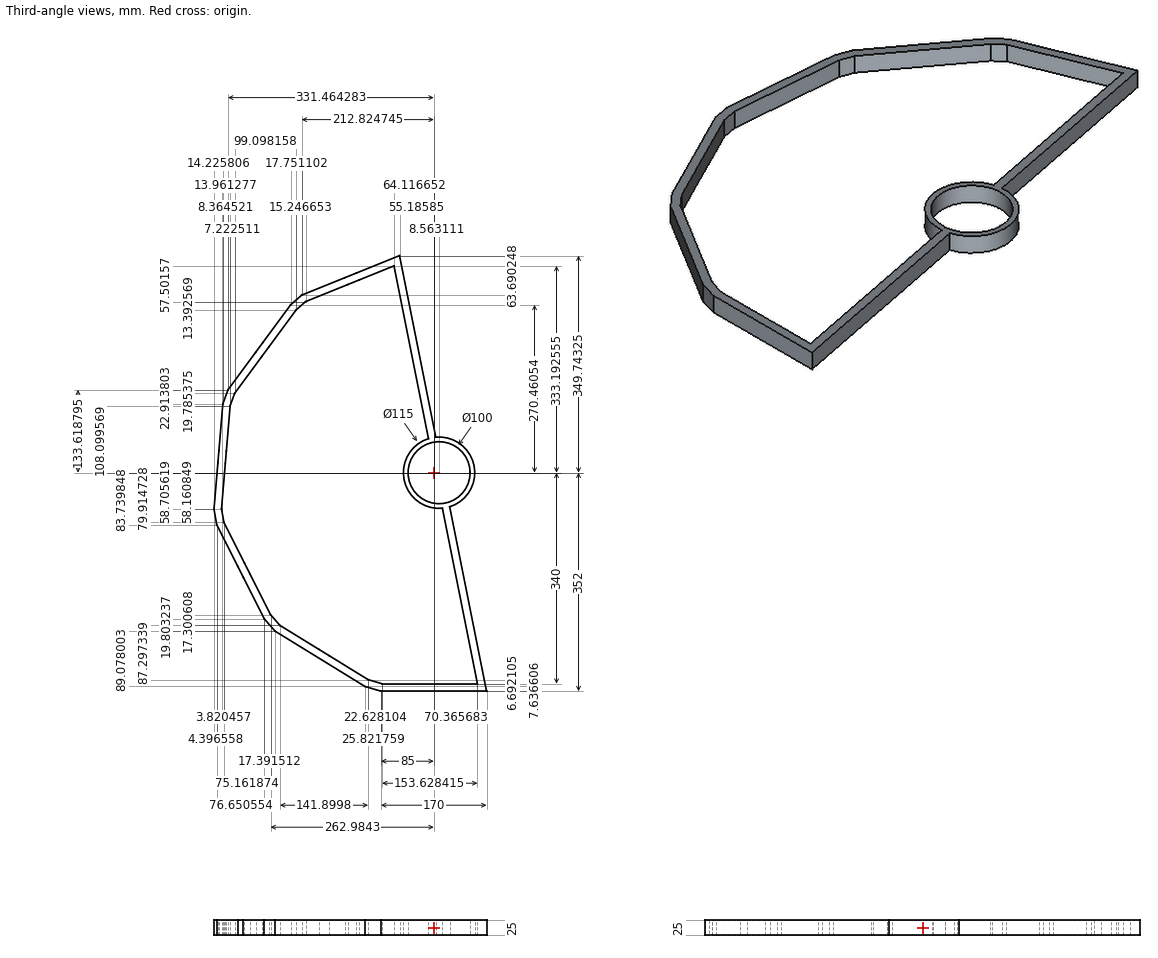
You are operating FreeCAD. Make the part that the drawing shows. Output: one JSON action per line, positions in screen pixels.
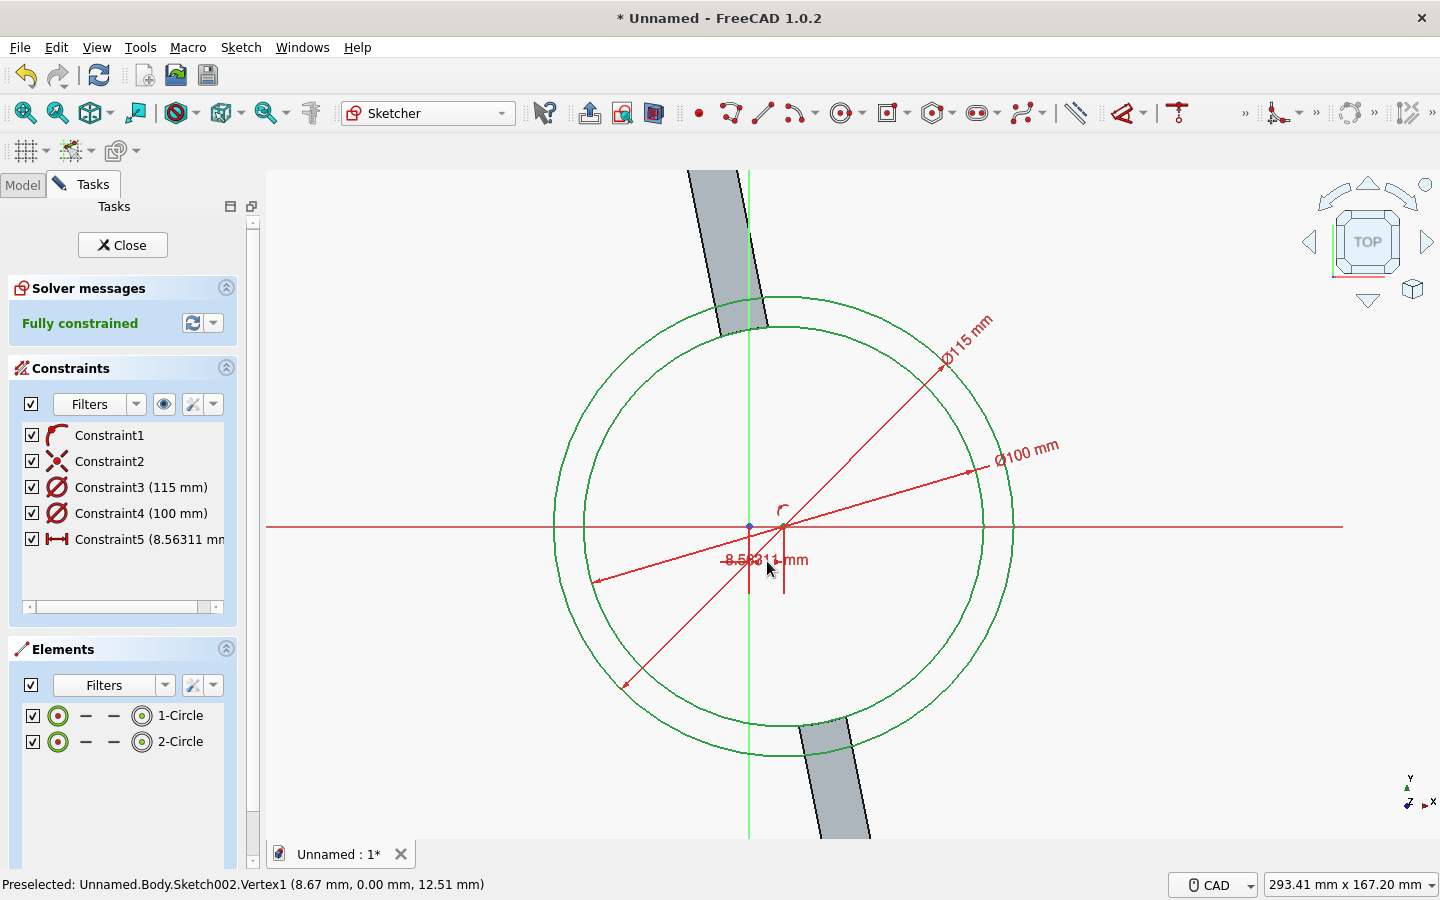
{"action": "left_click", "coordinate": [123, 245]}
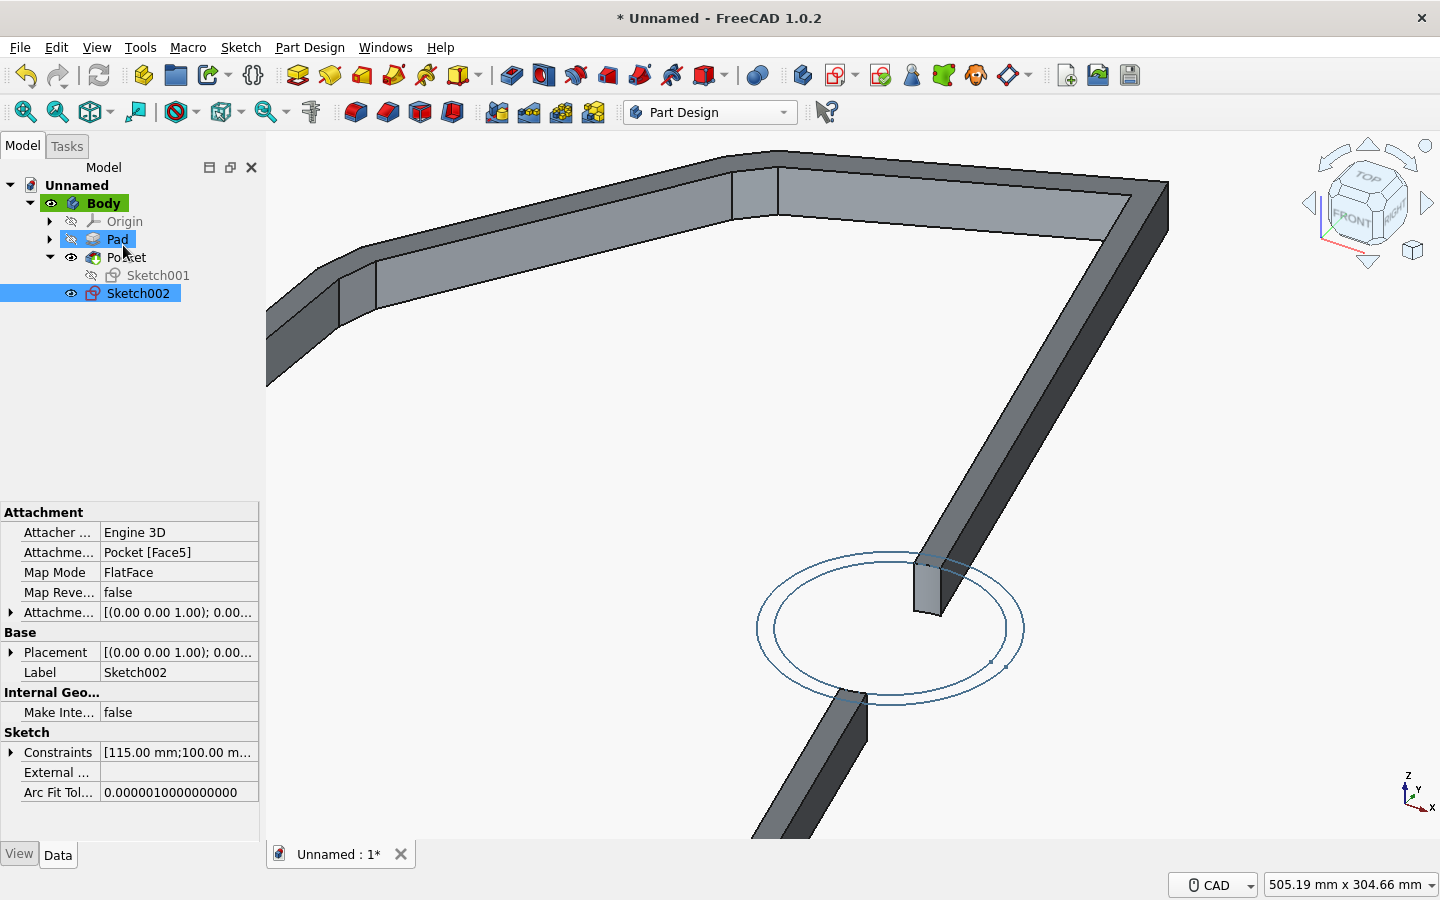
{"action": "left_click", "coordinate": [298, 76]}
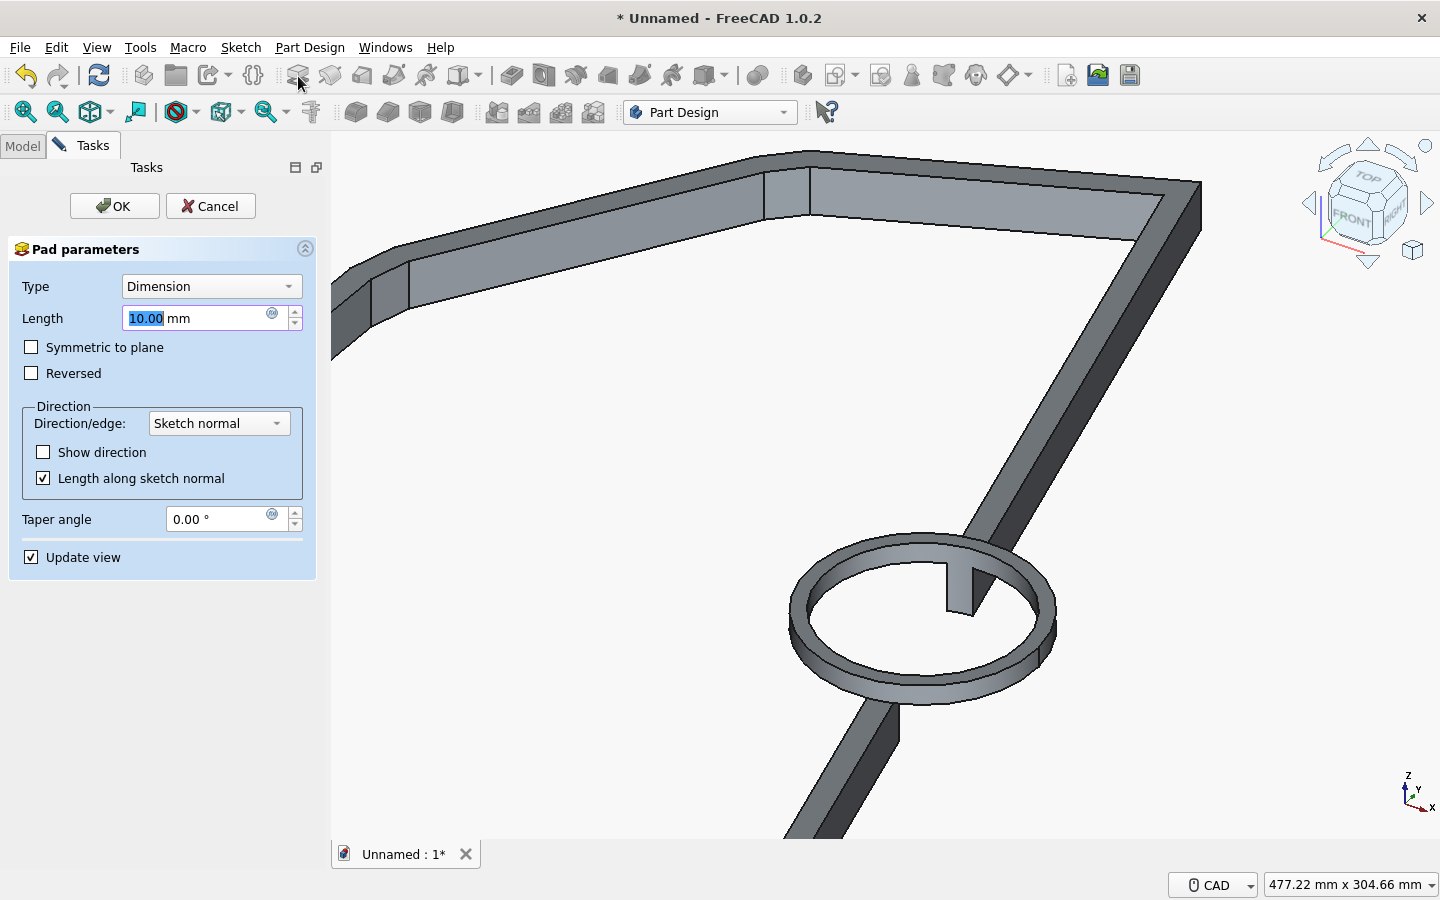
{"action": "type", "text": "25"}
{"action": "key", "text": "Tab"}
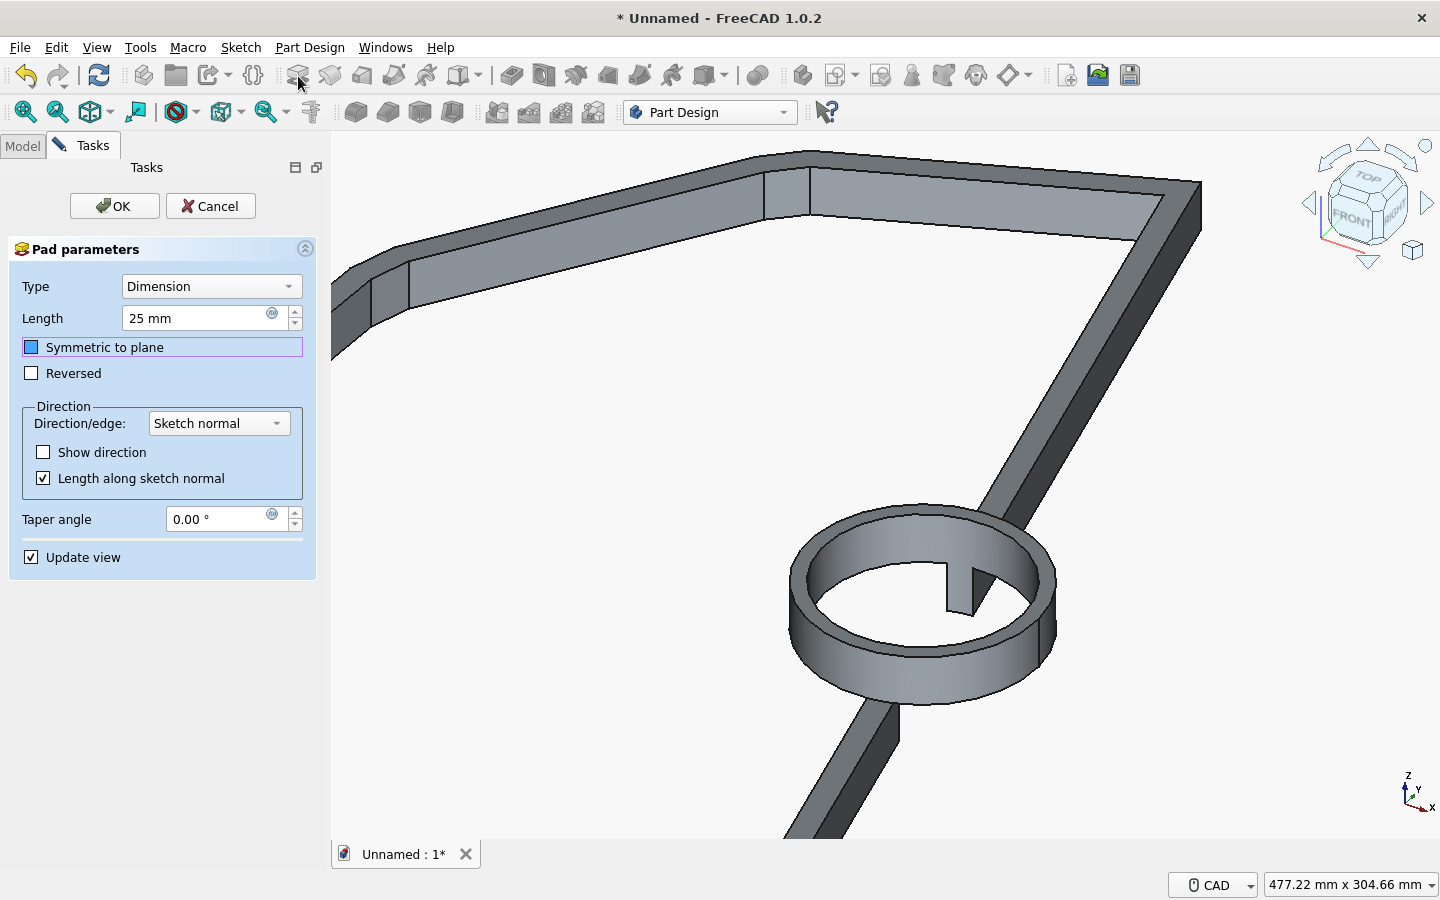
{"action": "left_click", "coordinate": [30, 373]}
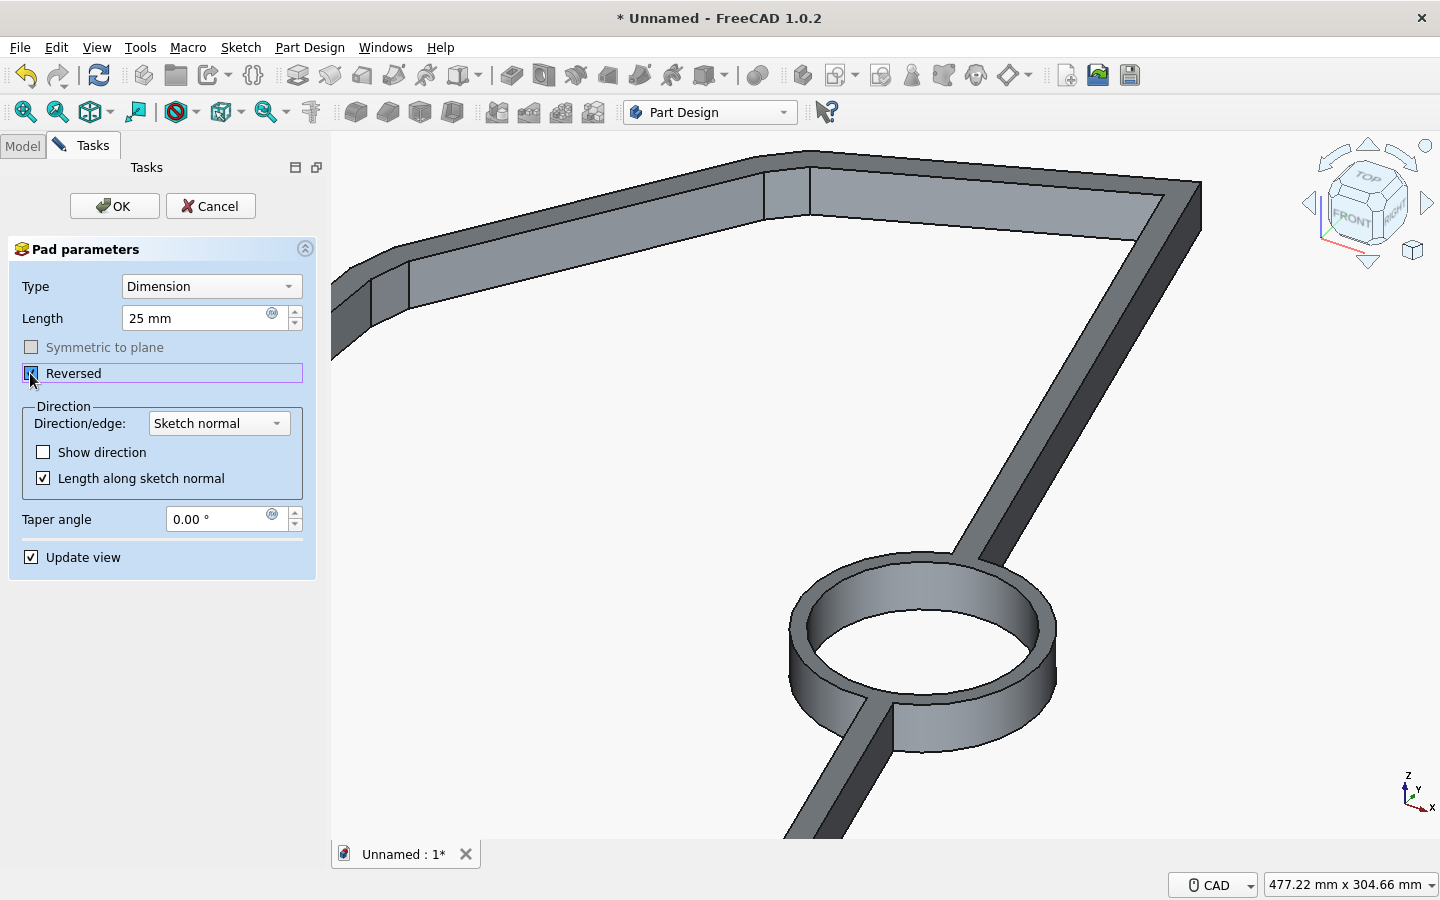
{"action": "left_click", "coordinate": [115, 206]}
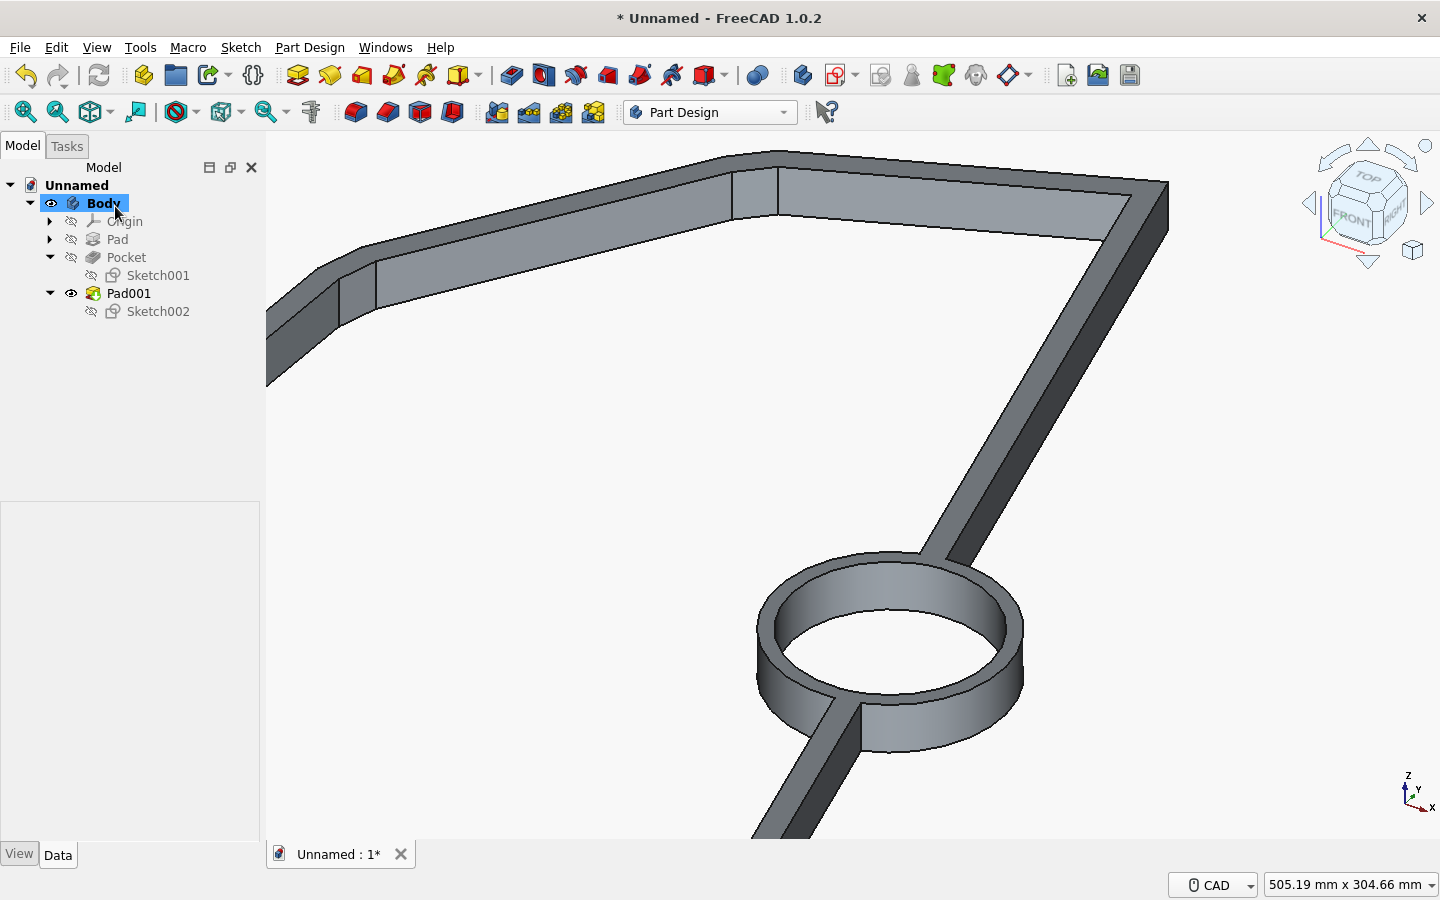
{"action": "key", "text": "0"}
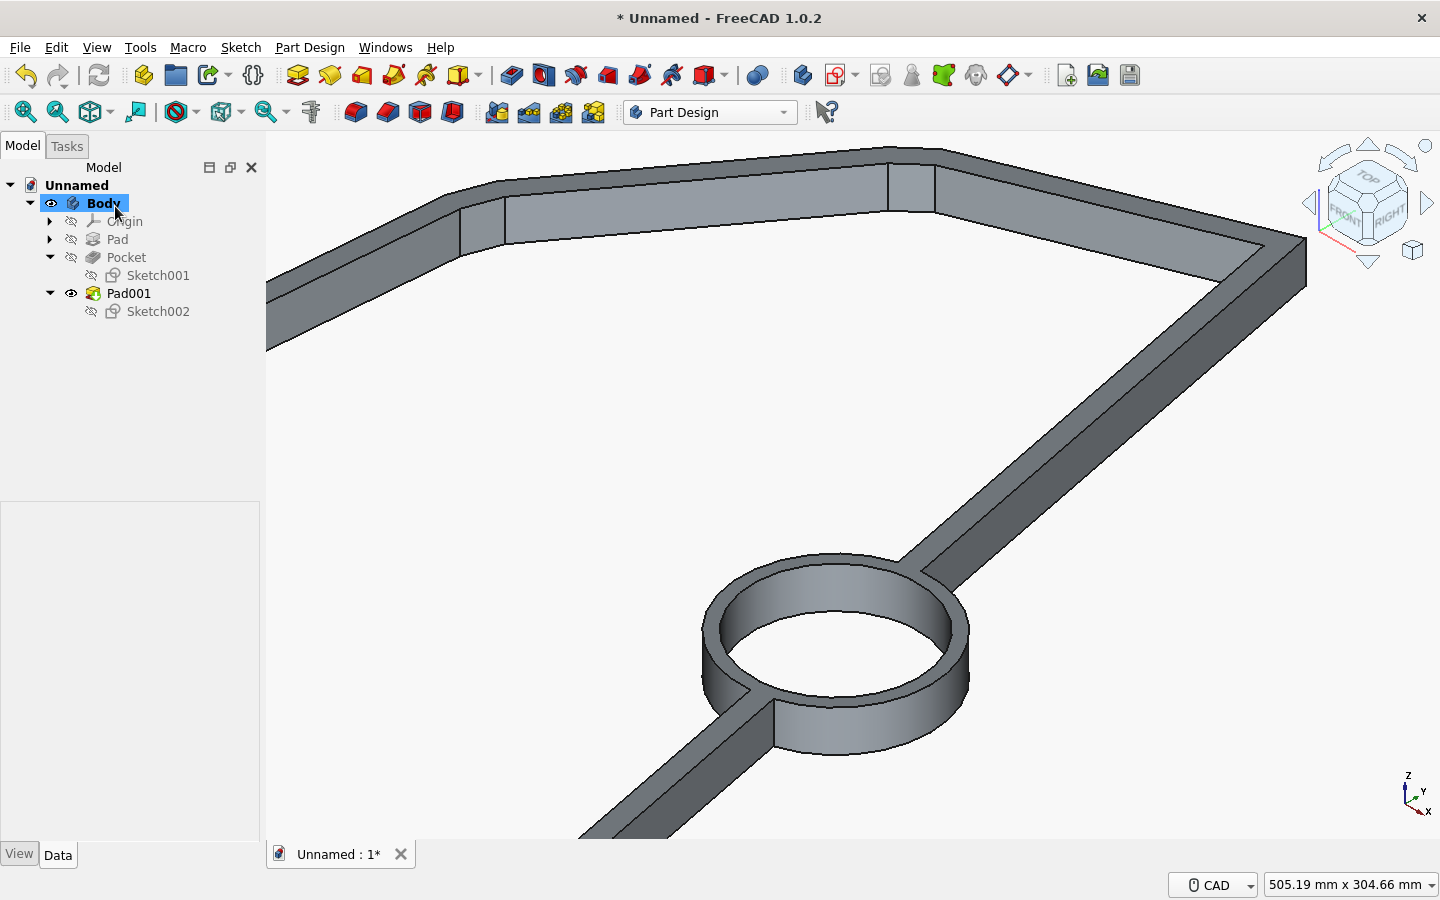
{"action": "left_click", "coordinate": [26, 112]}